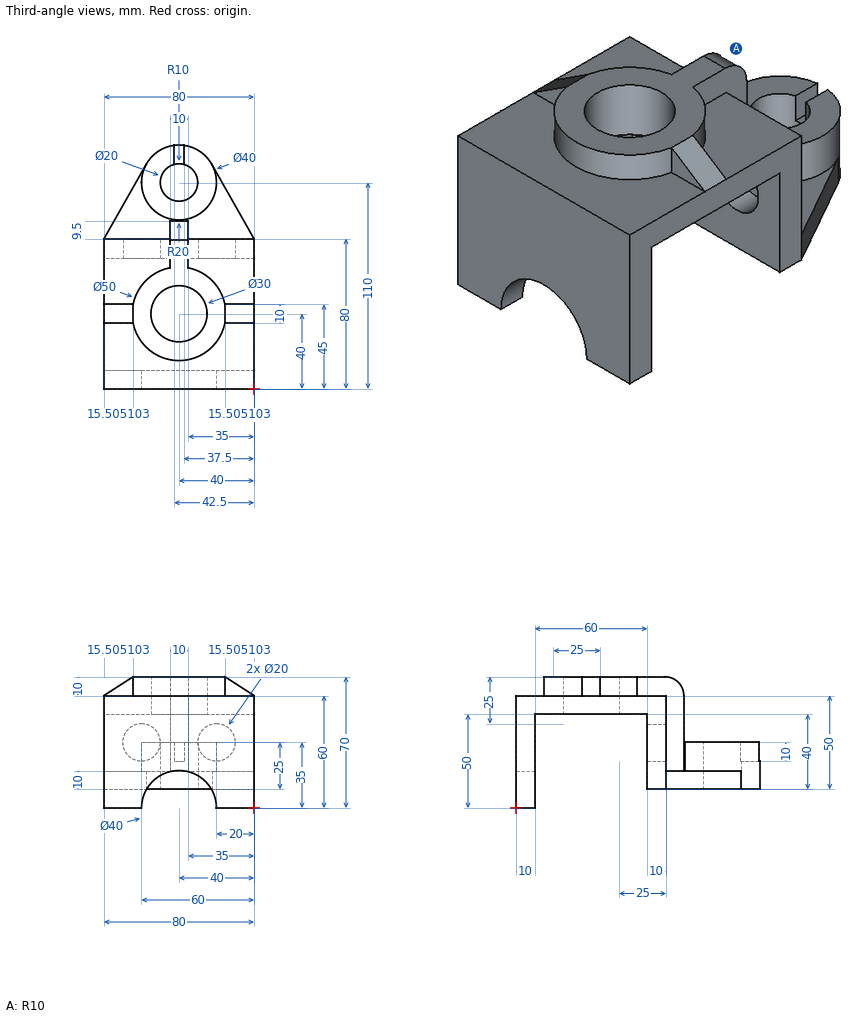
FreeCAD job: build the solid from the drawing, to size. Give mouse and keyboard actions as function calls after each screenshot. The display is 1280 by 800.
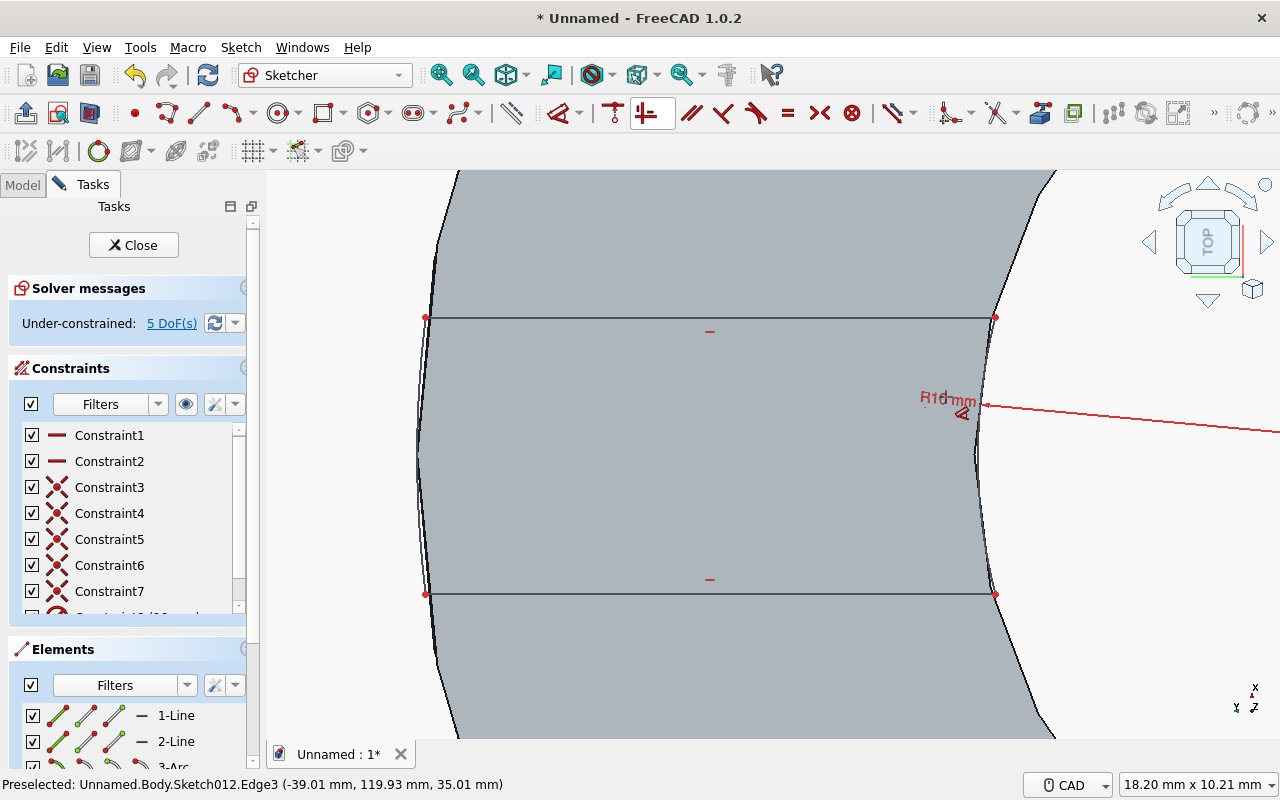
click(419, 400)
click(387, 398)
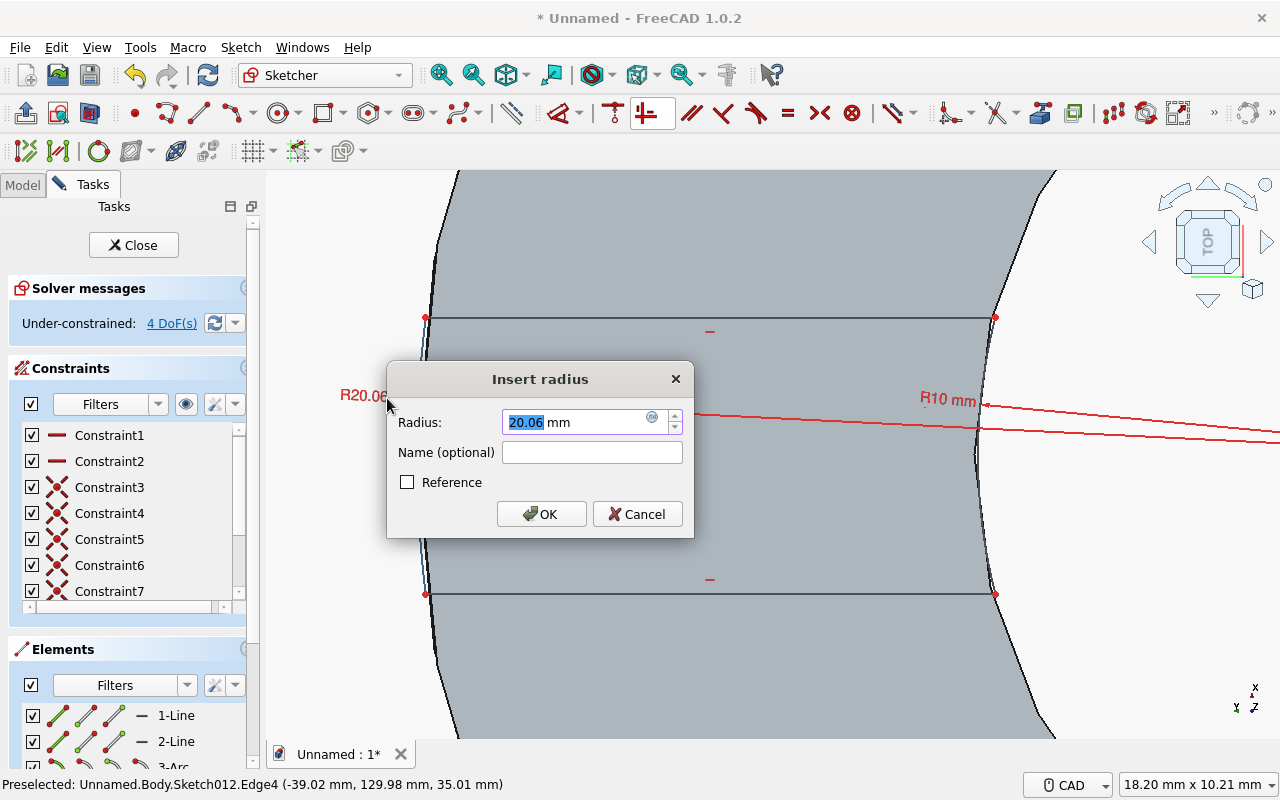
text(20)
key(Return)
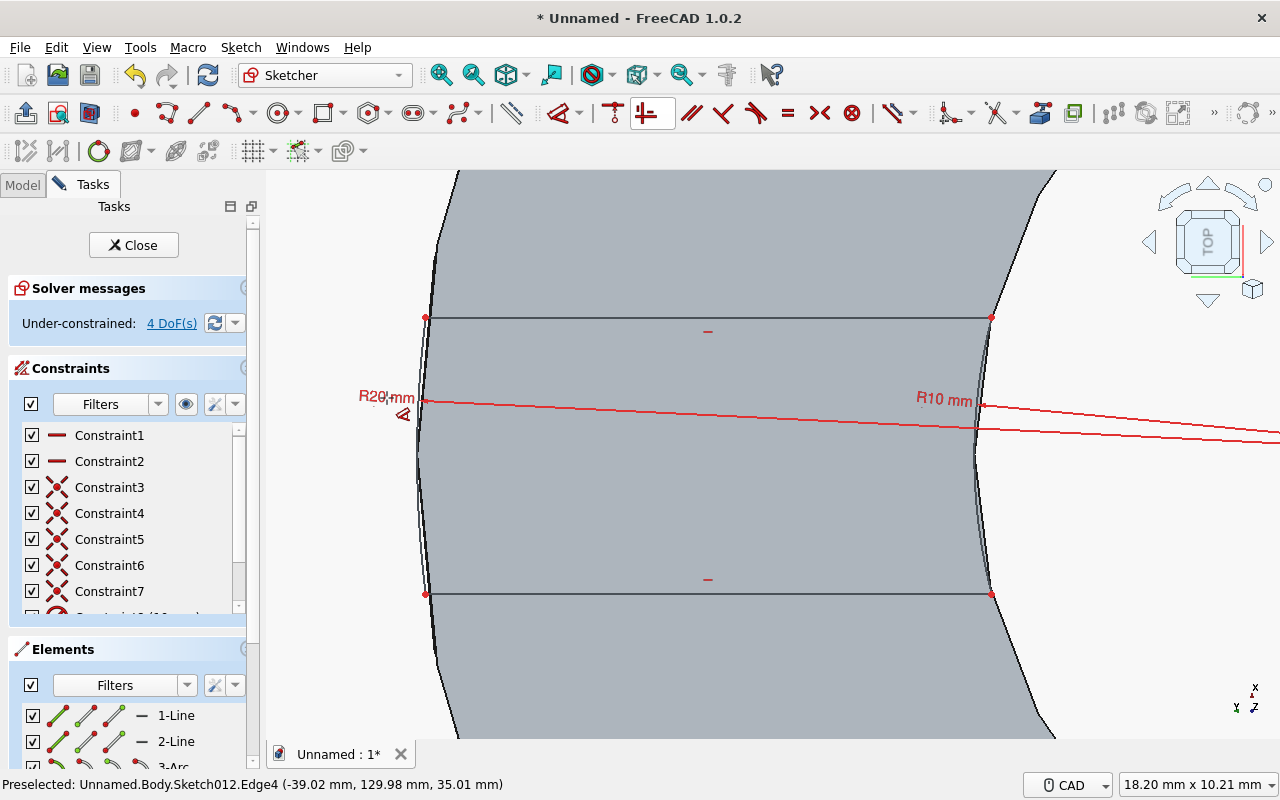
scroll(376, 454, down, 3)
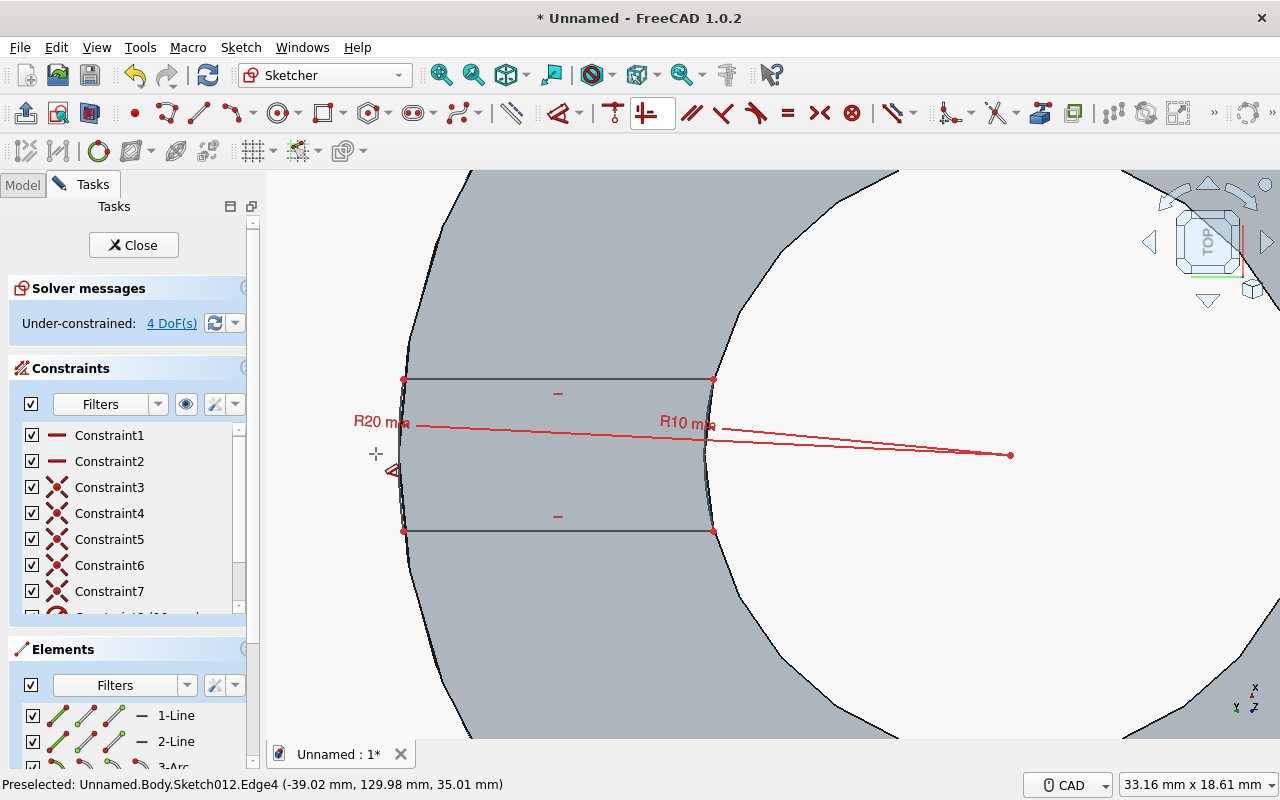
click(1010, 455)
click(976, 327)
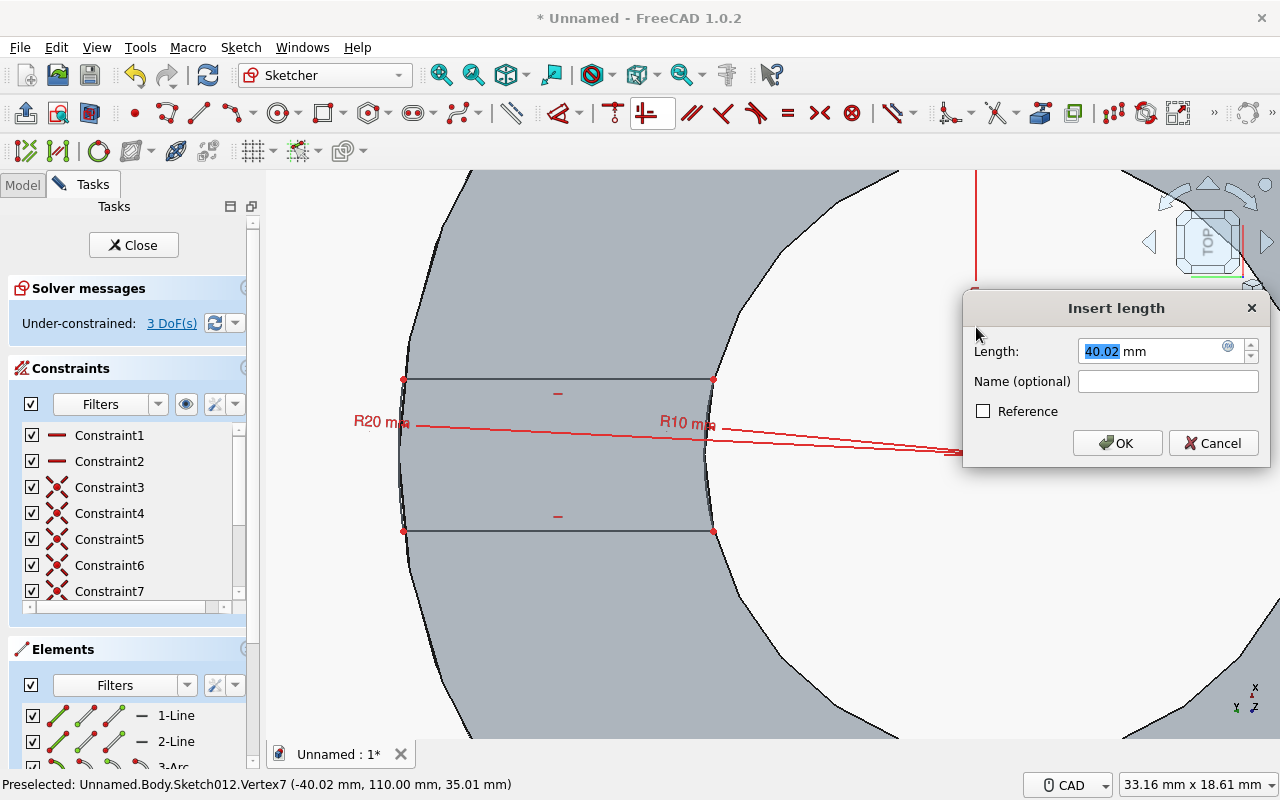
text(40)
key(Return)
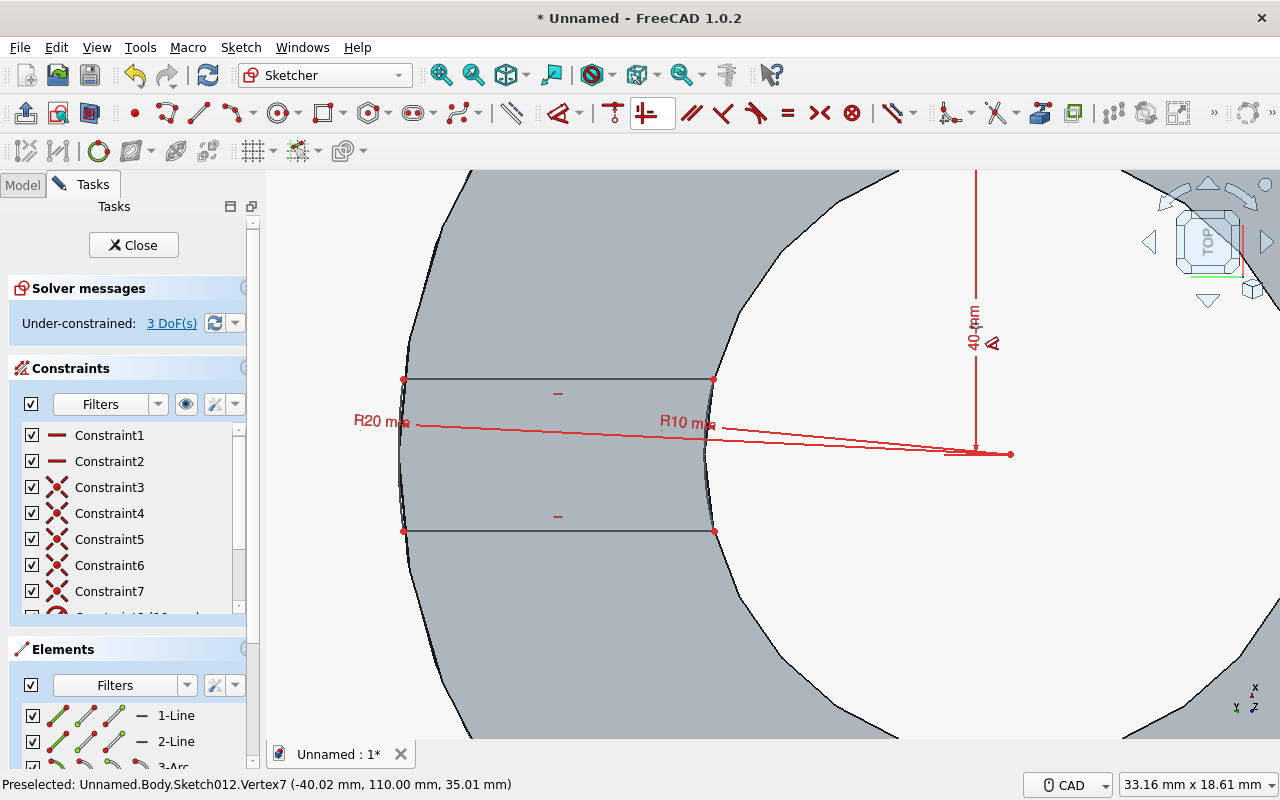
click(1010, 455)
click(1063, 489)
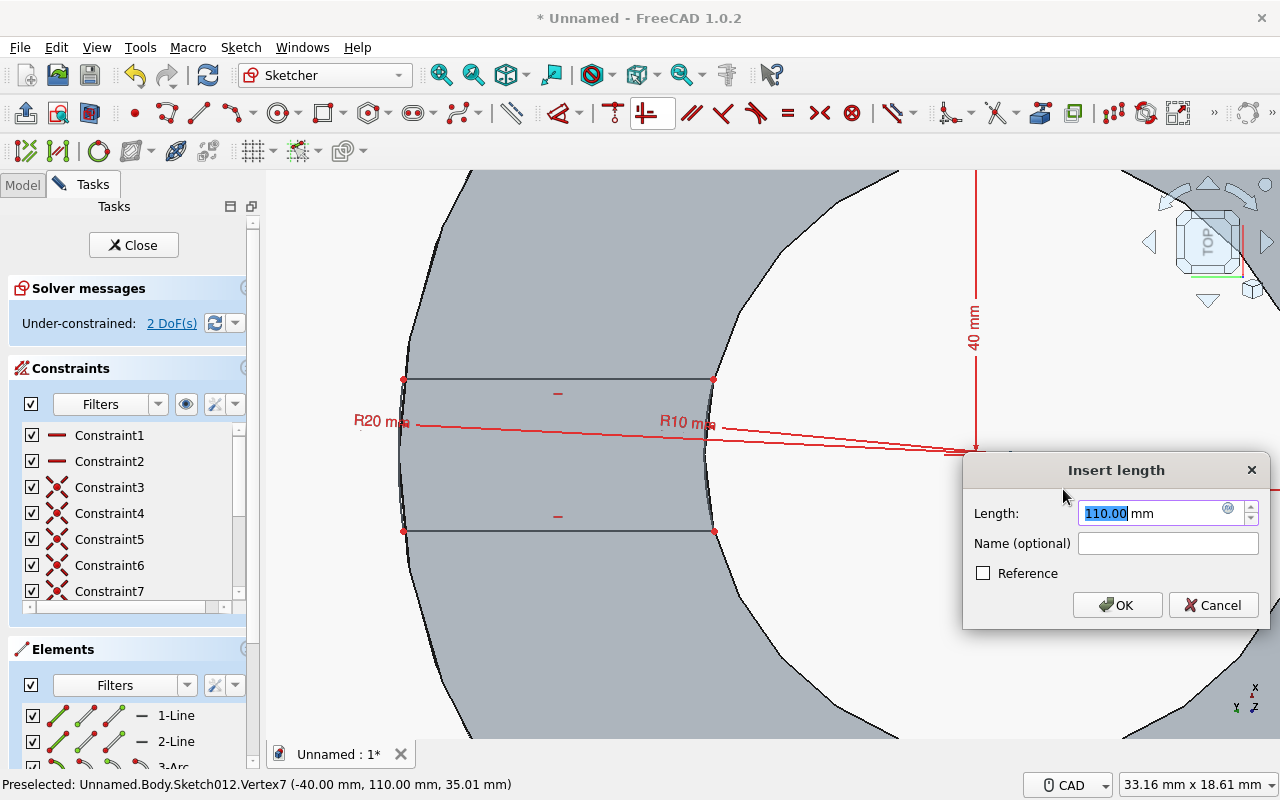
text(110)
key(Return)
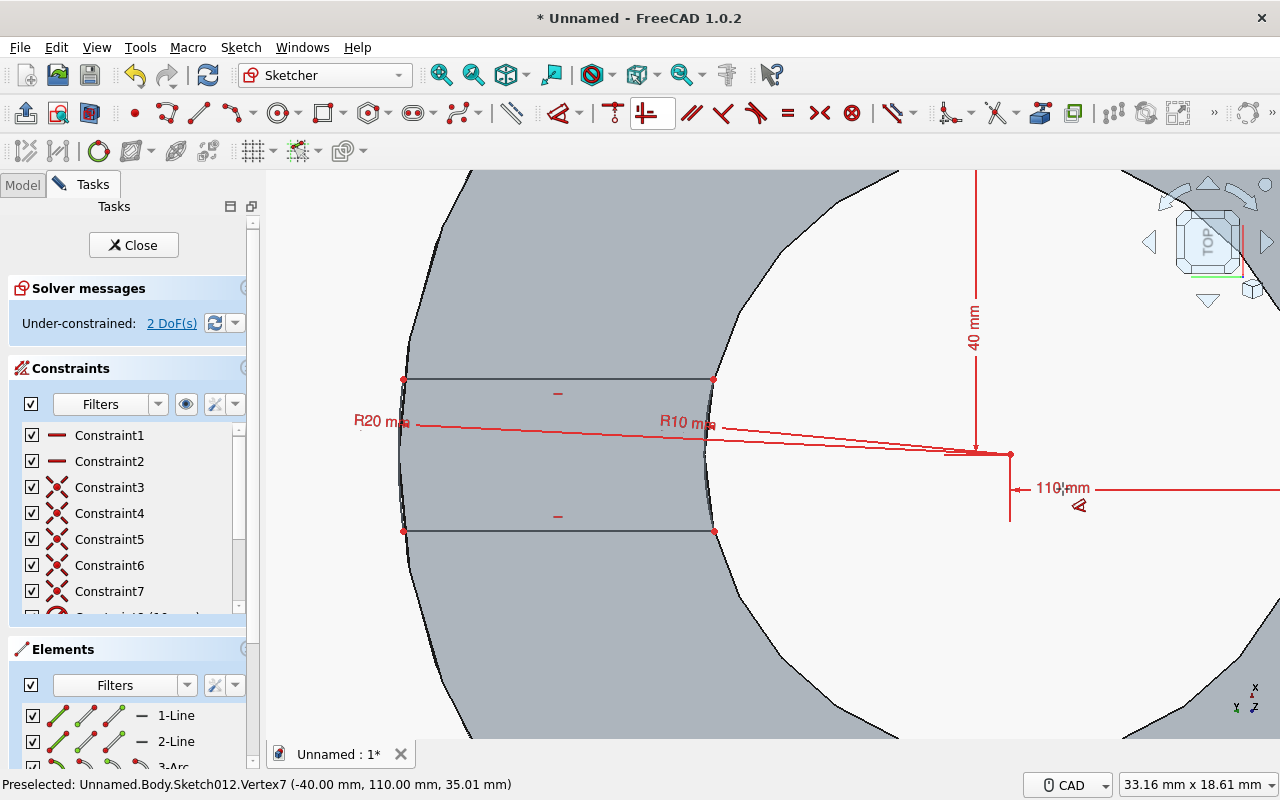
click(403, 531)
click(369, 365)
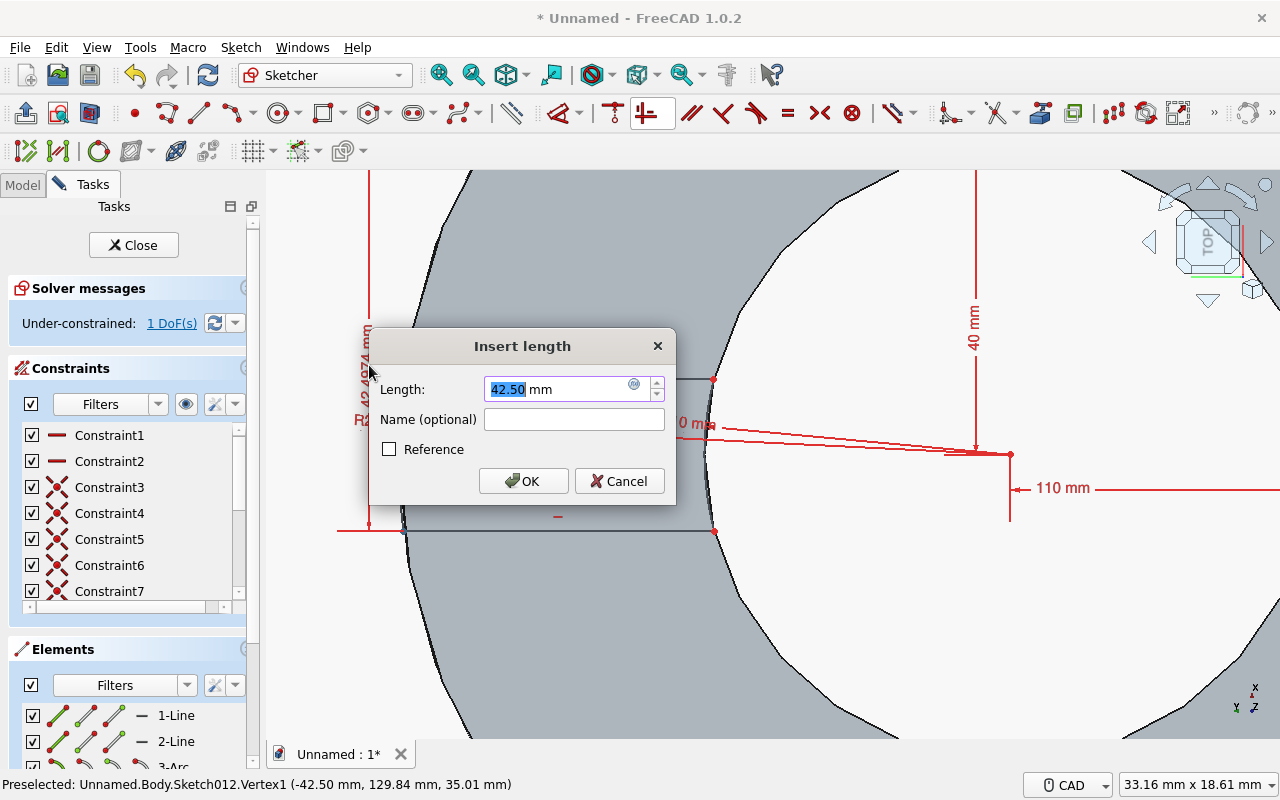
text(42.5)
key(Return)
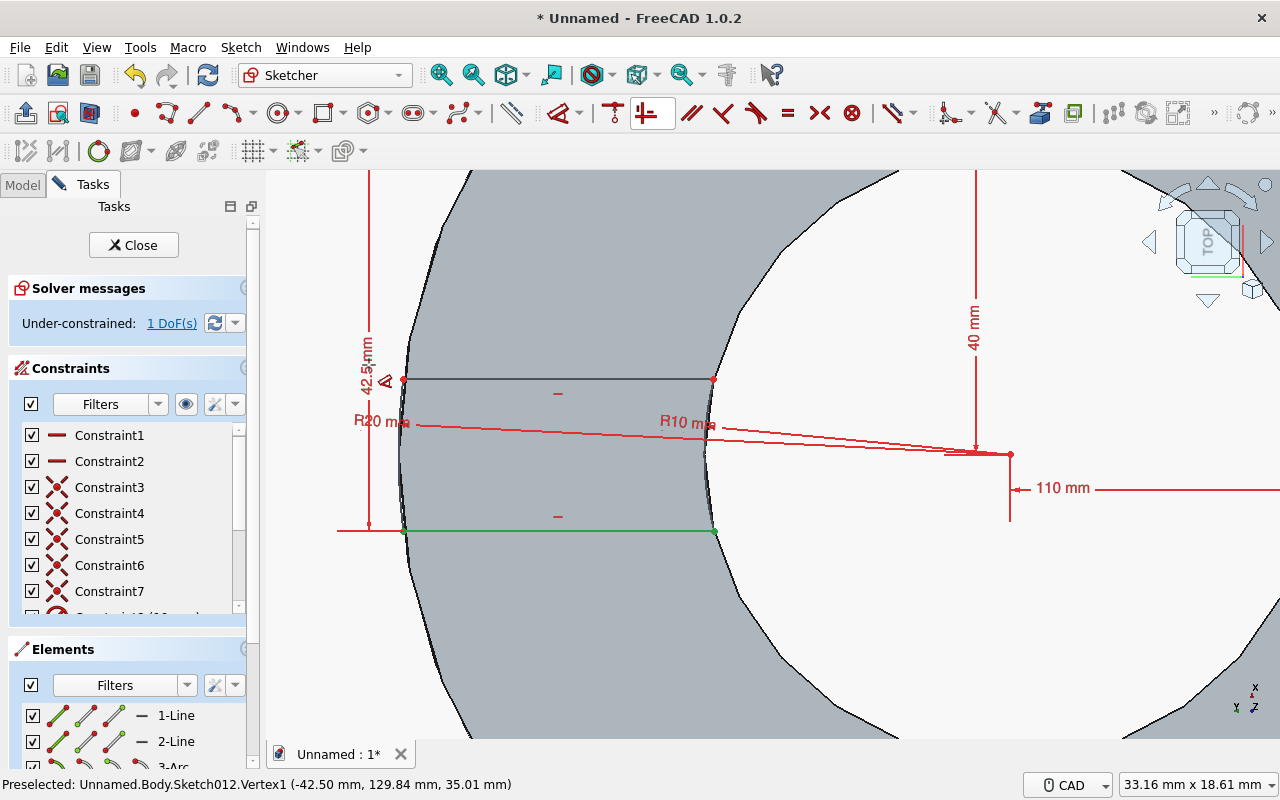
click(714, 379)
click(680, 289)